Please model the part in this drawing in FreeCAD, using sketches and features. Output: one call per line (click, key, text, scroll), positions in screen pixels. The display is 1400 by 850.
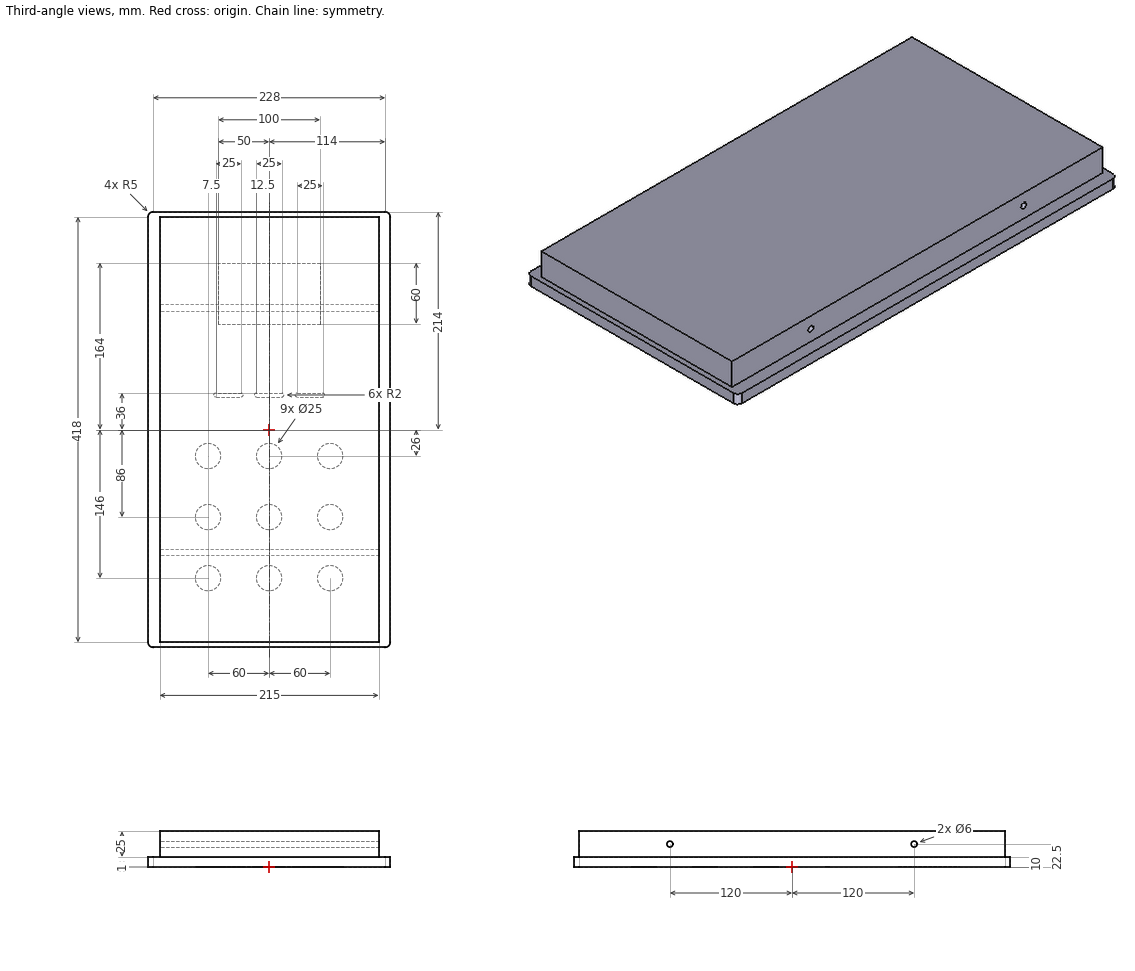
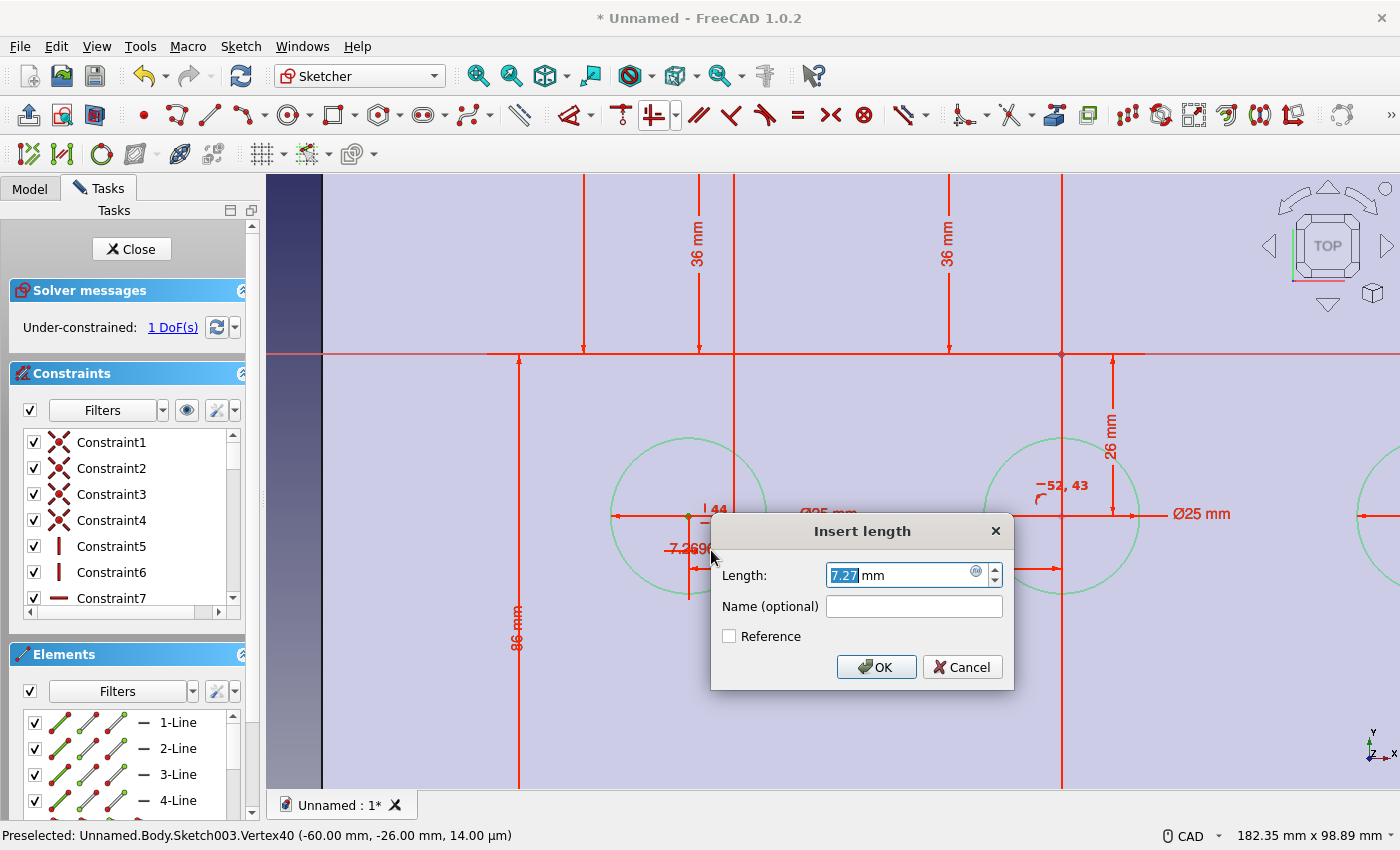
text(7.5)
key(Return)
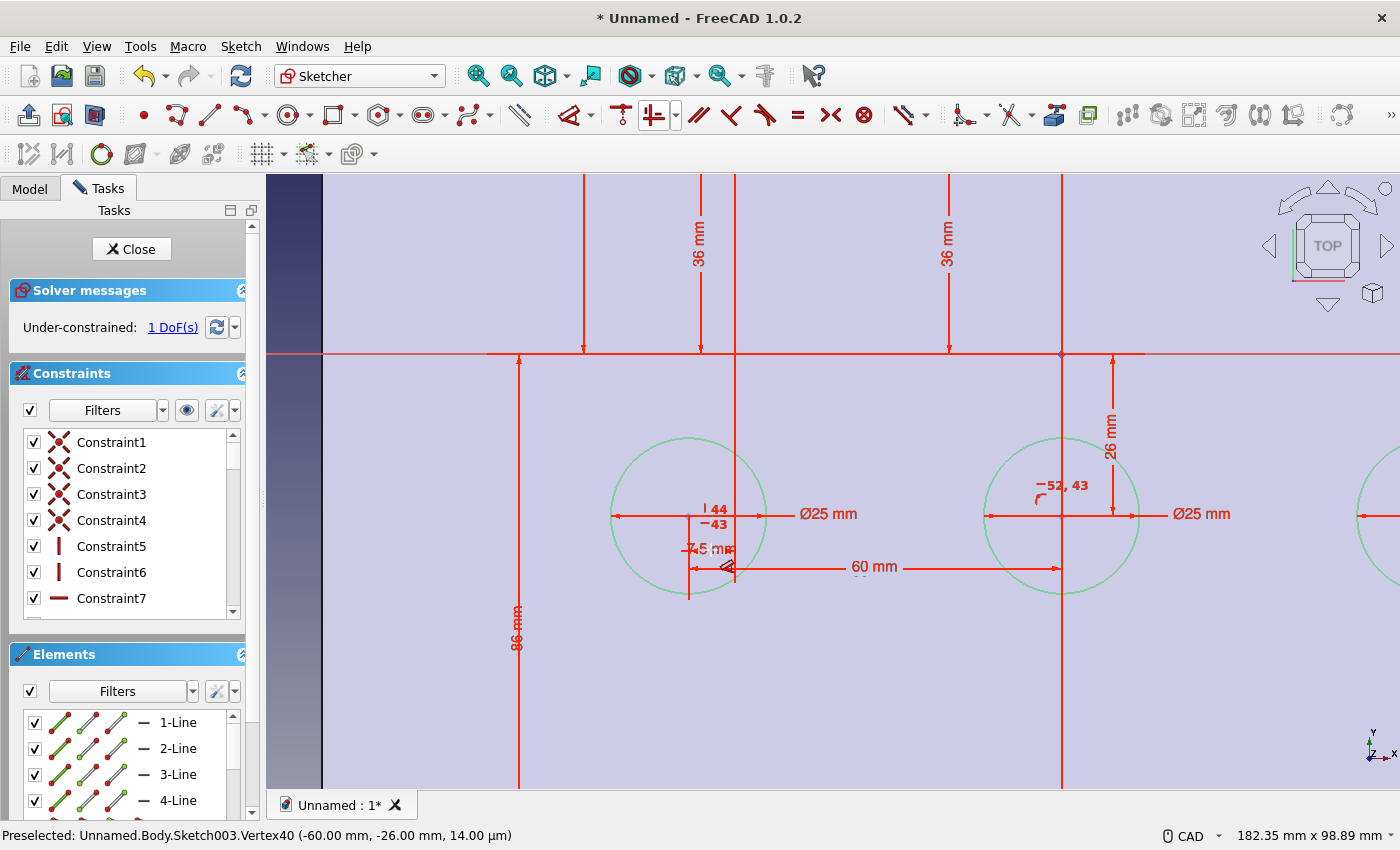
scroll(689, 518, down, 8)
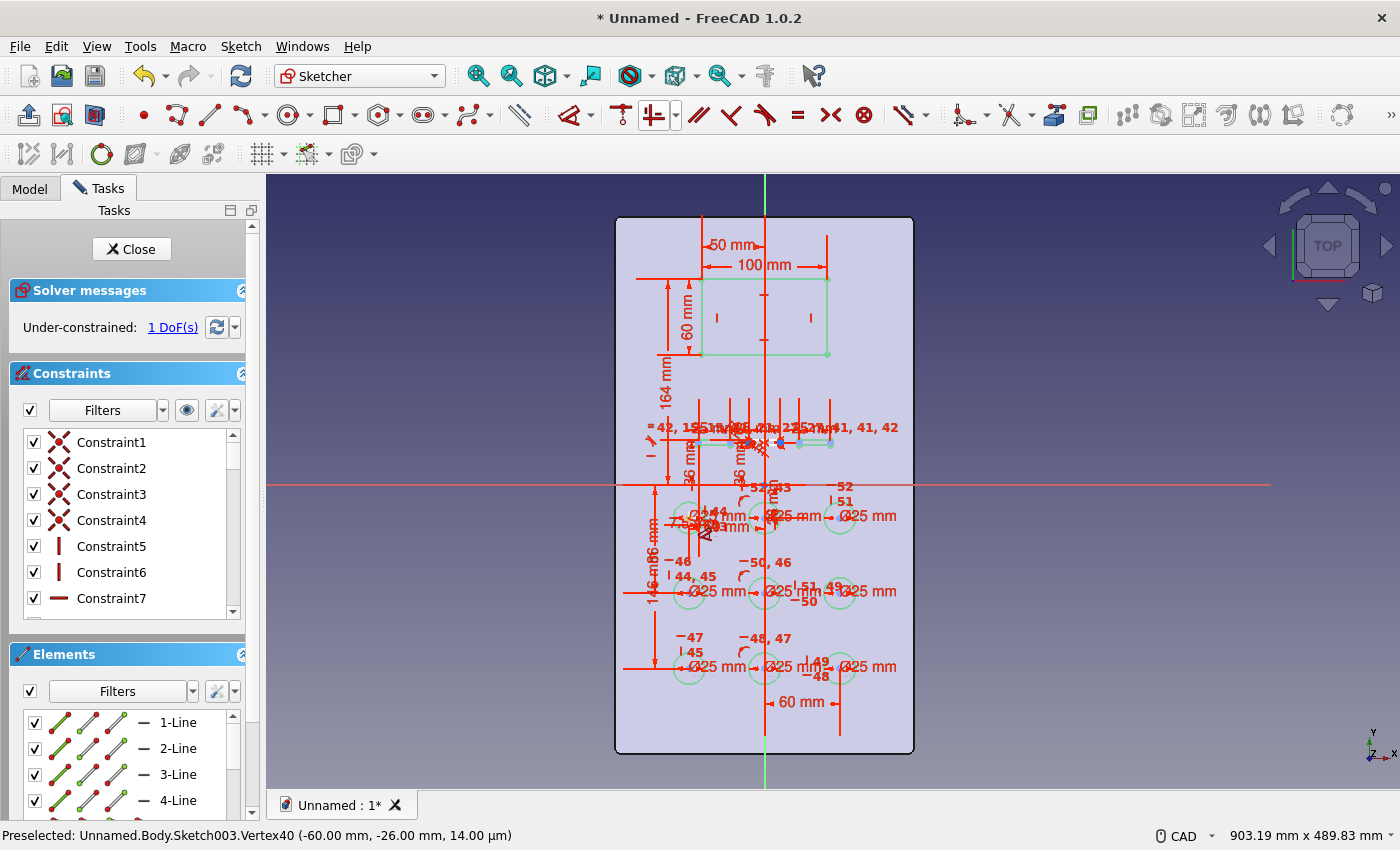
scroll(749, 440, up, 8)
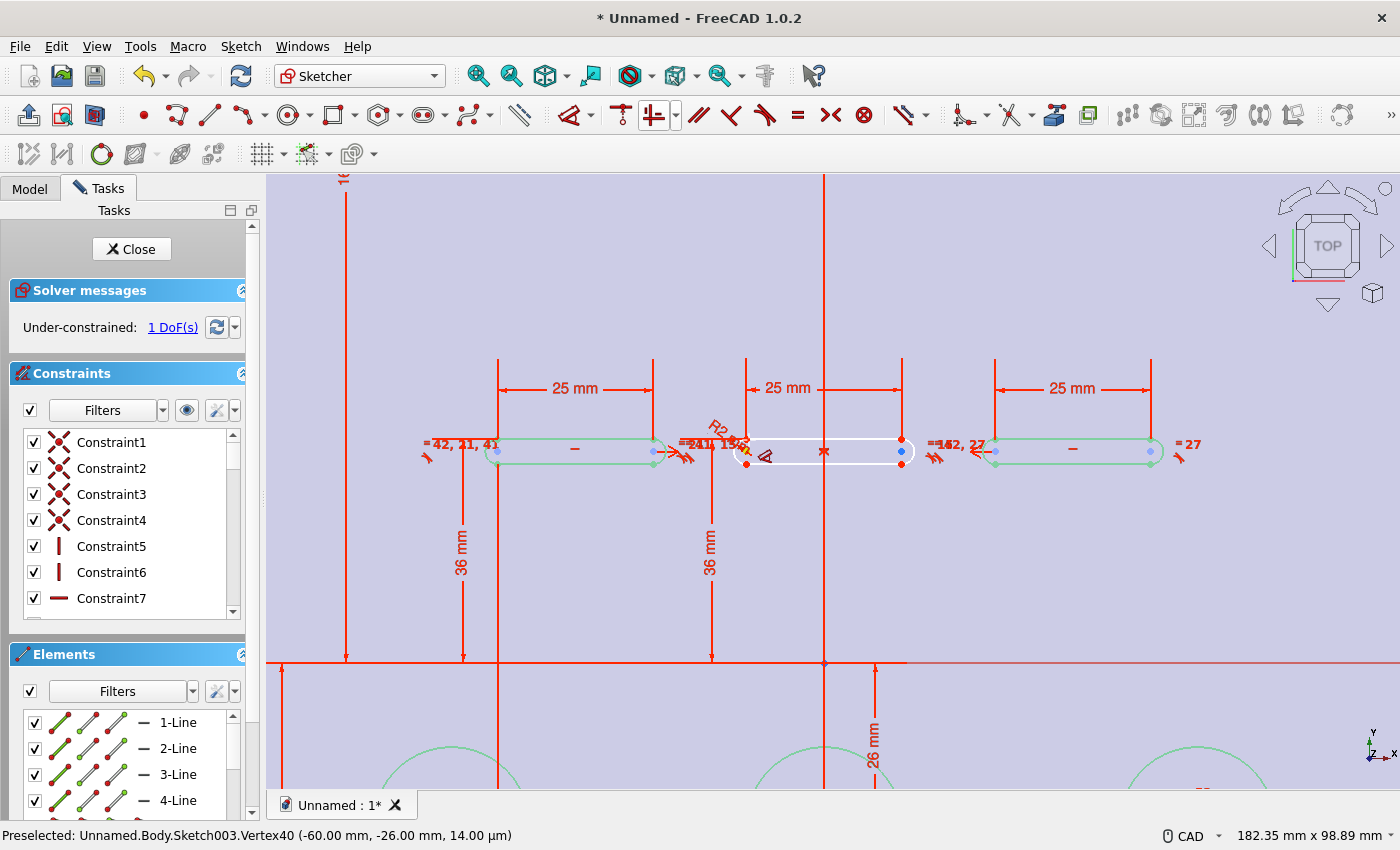
click(746, 439)
click(785, 697)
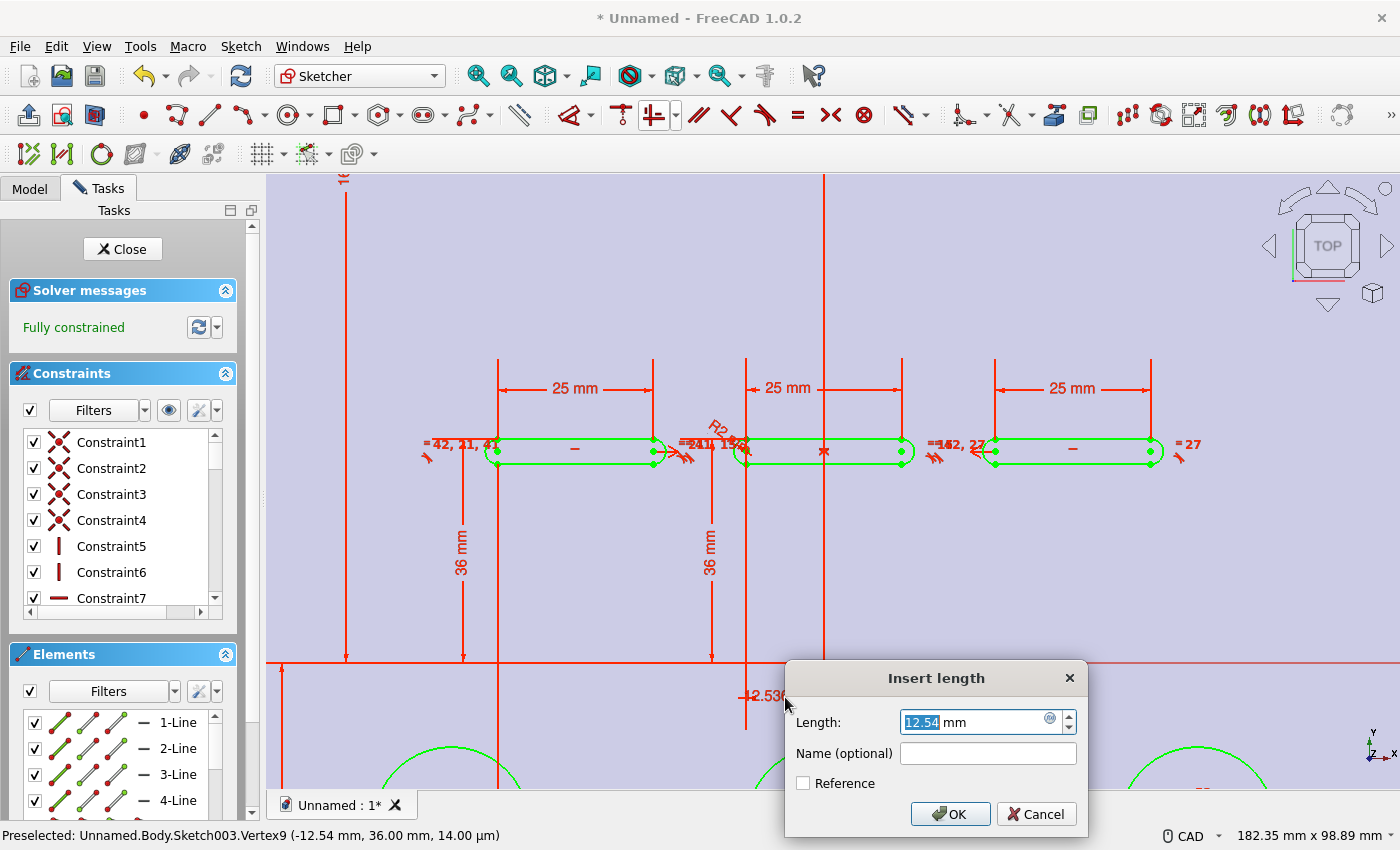
text(12.5)
key(Return)
key(Escape)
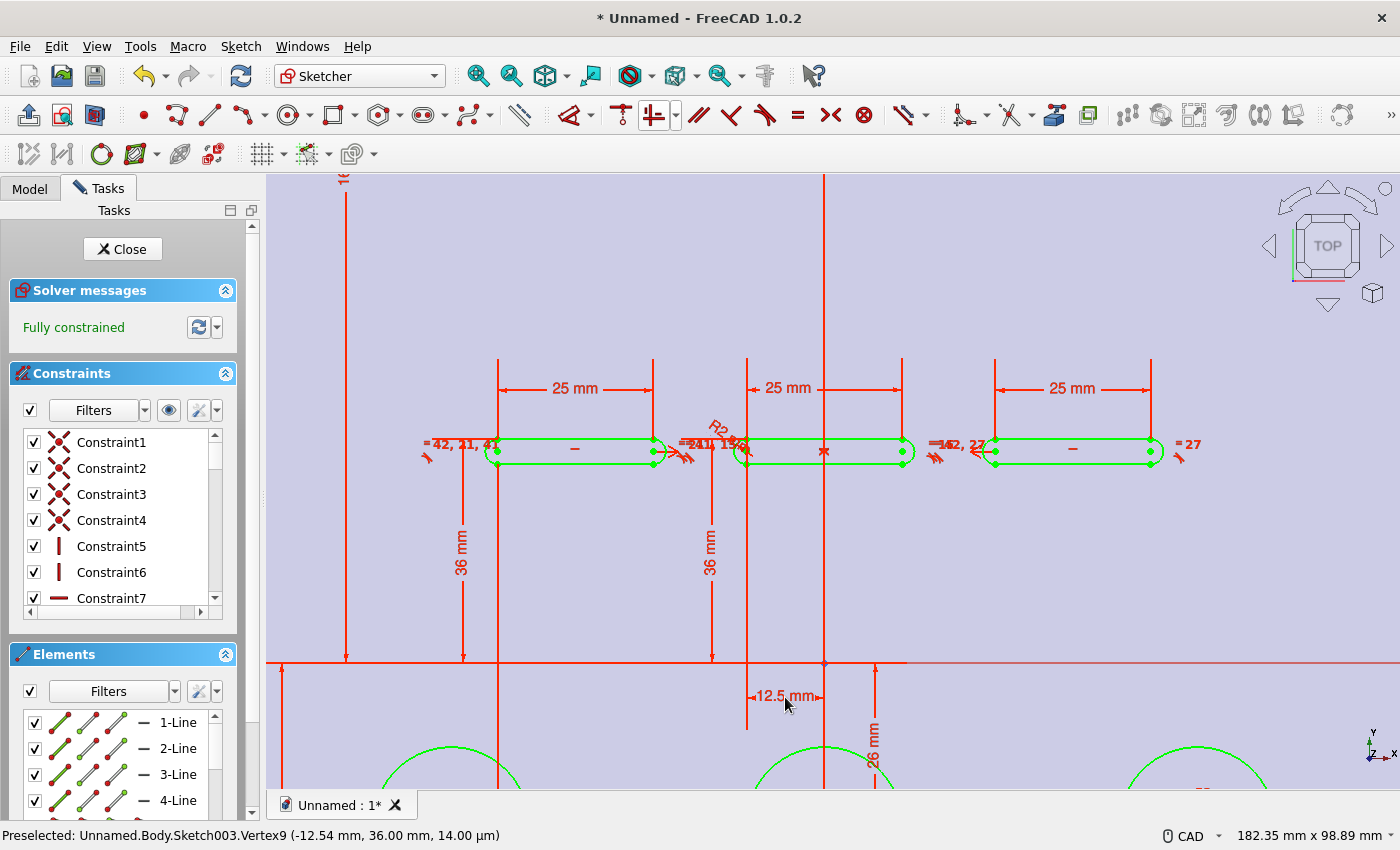
click(123, 249)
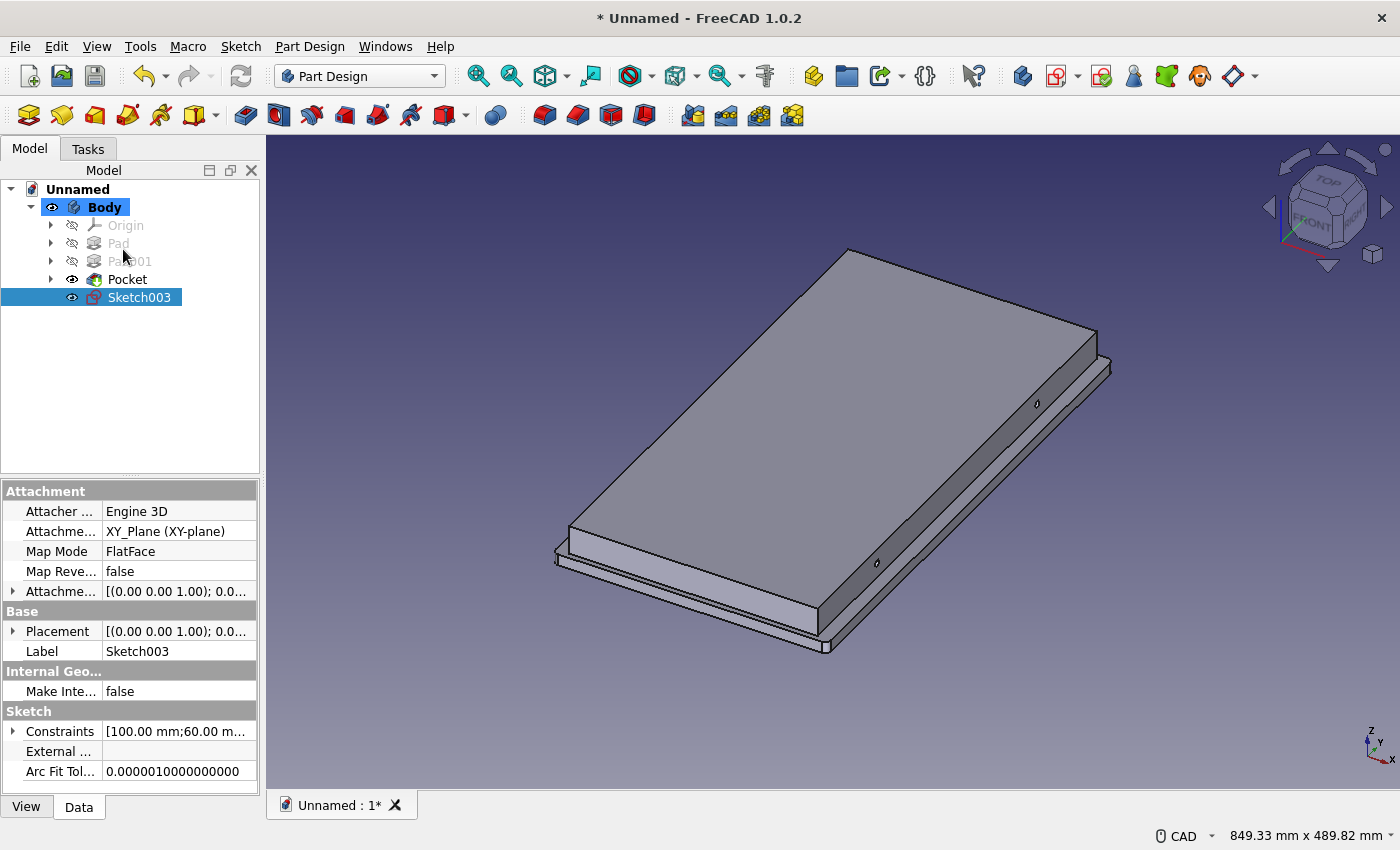
click(246, 116)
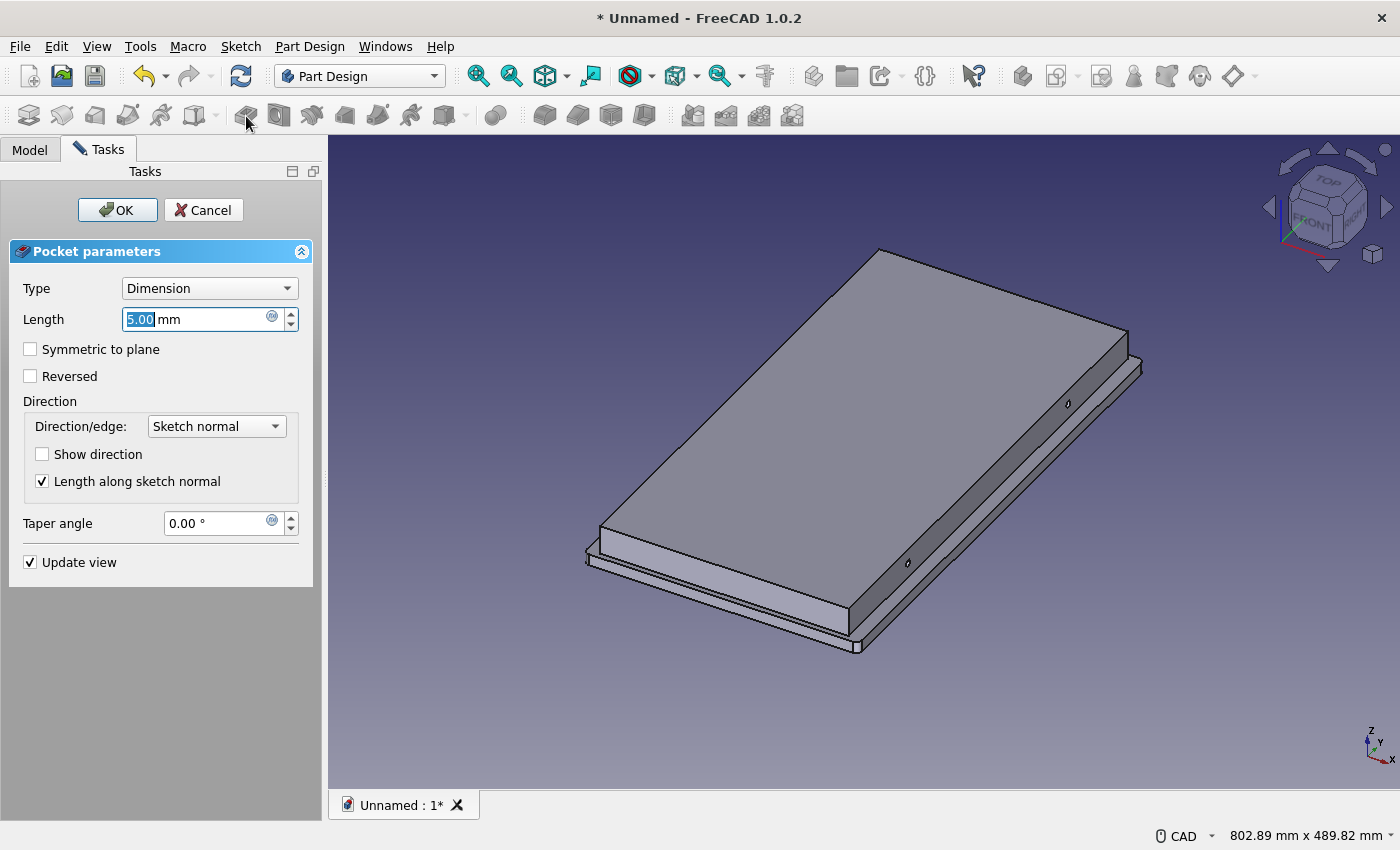
text(1)
key(Tab)